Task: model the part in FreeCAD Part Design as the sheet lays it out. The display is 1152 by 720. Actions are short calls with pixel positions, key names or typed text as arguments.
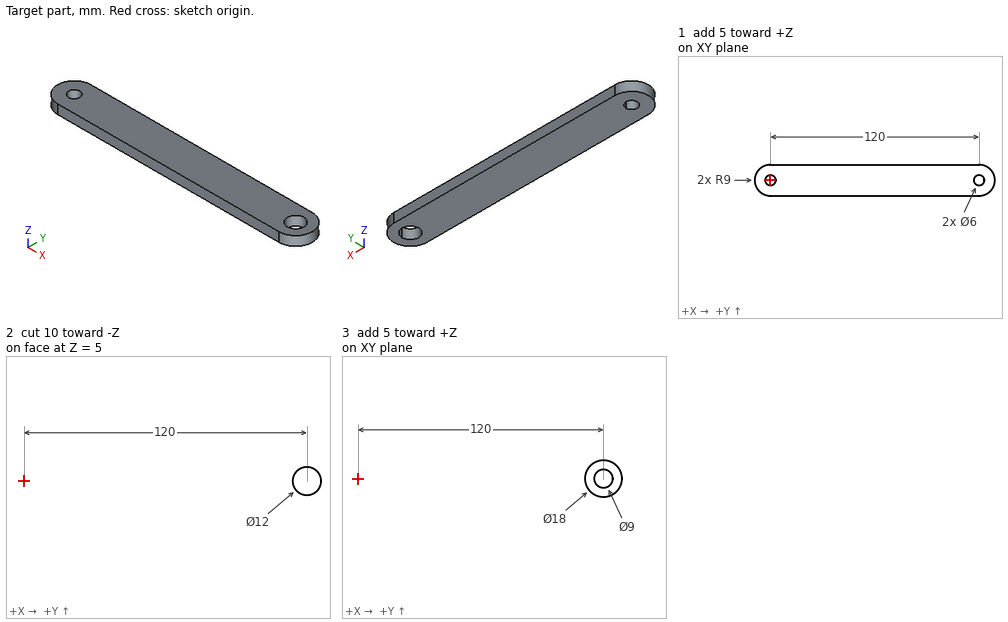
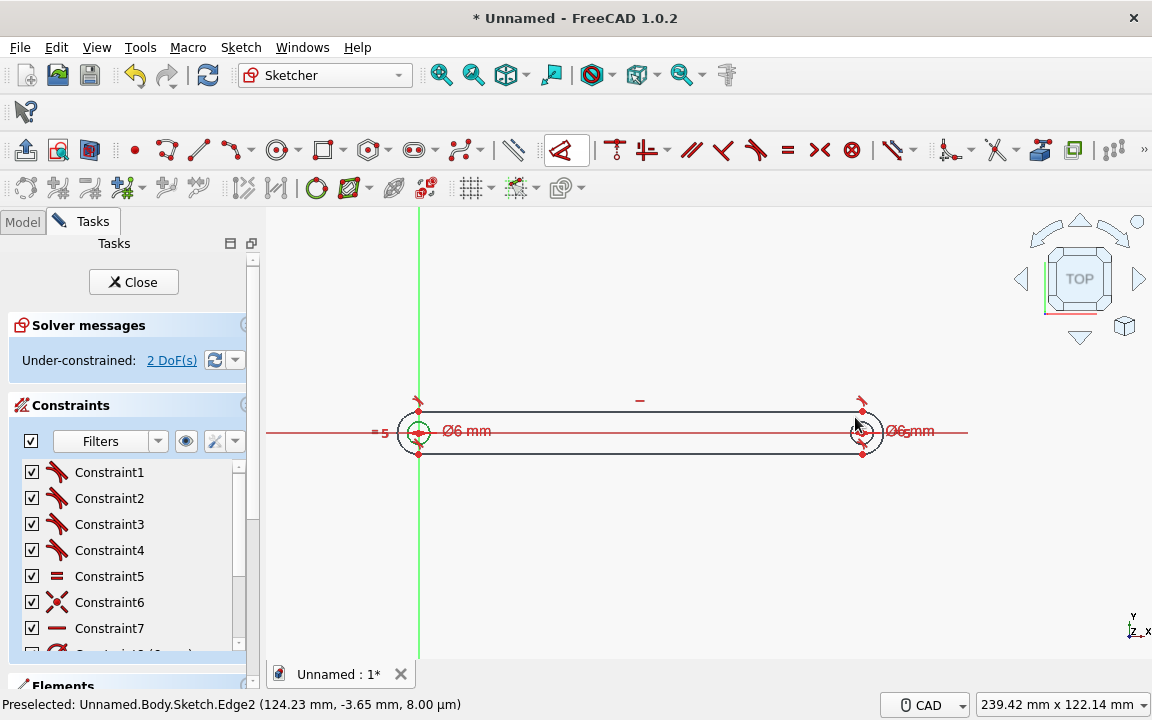
scroll(402, 421, up, 2)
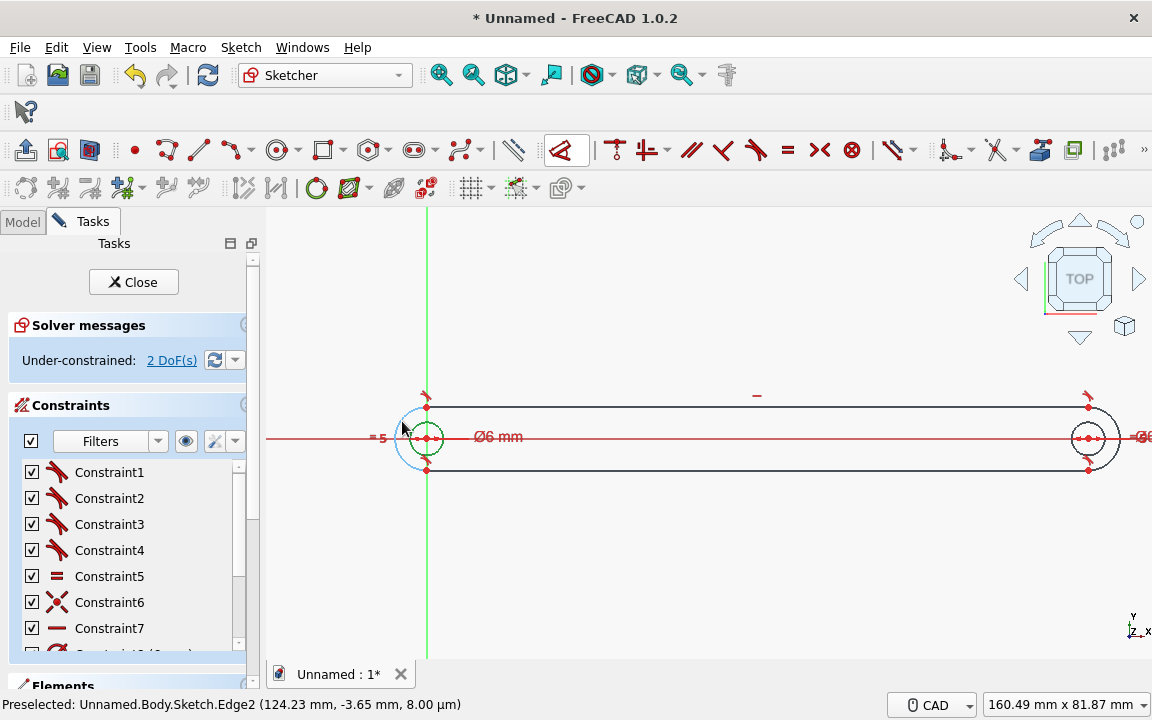
click(401, 420)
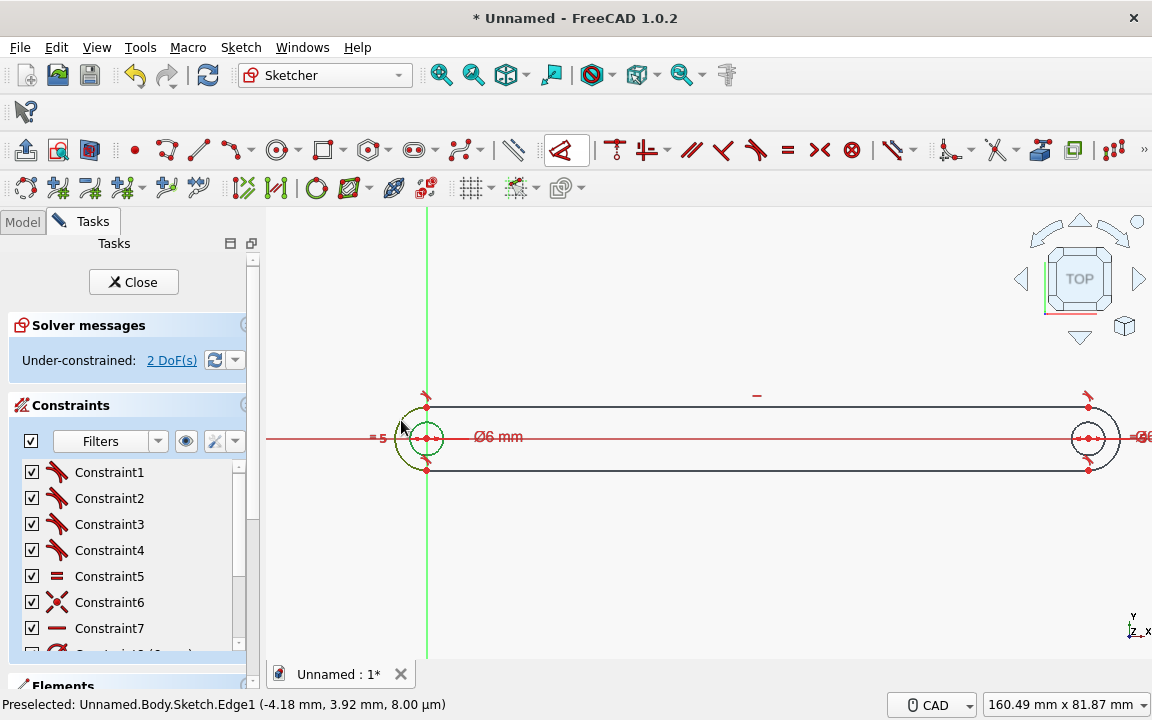
key(k)
key(r)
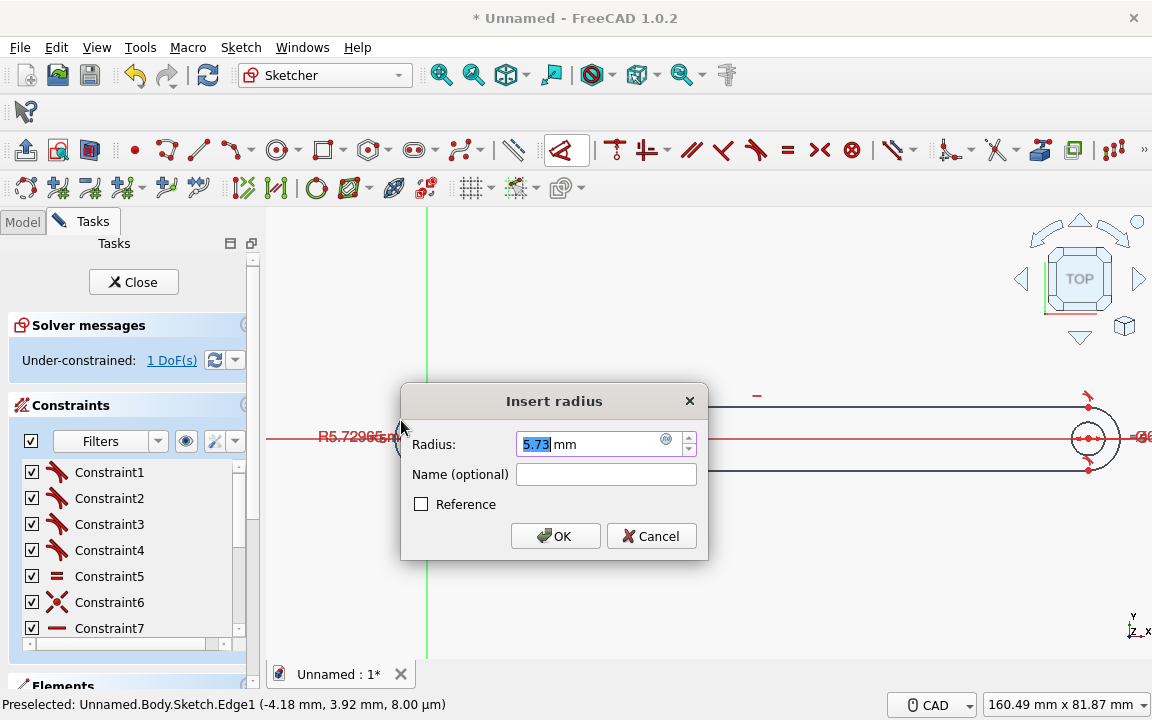
text(9)
key(Return)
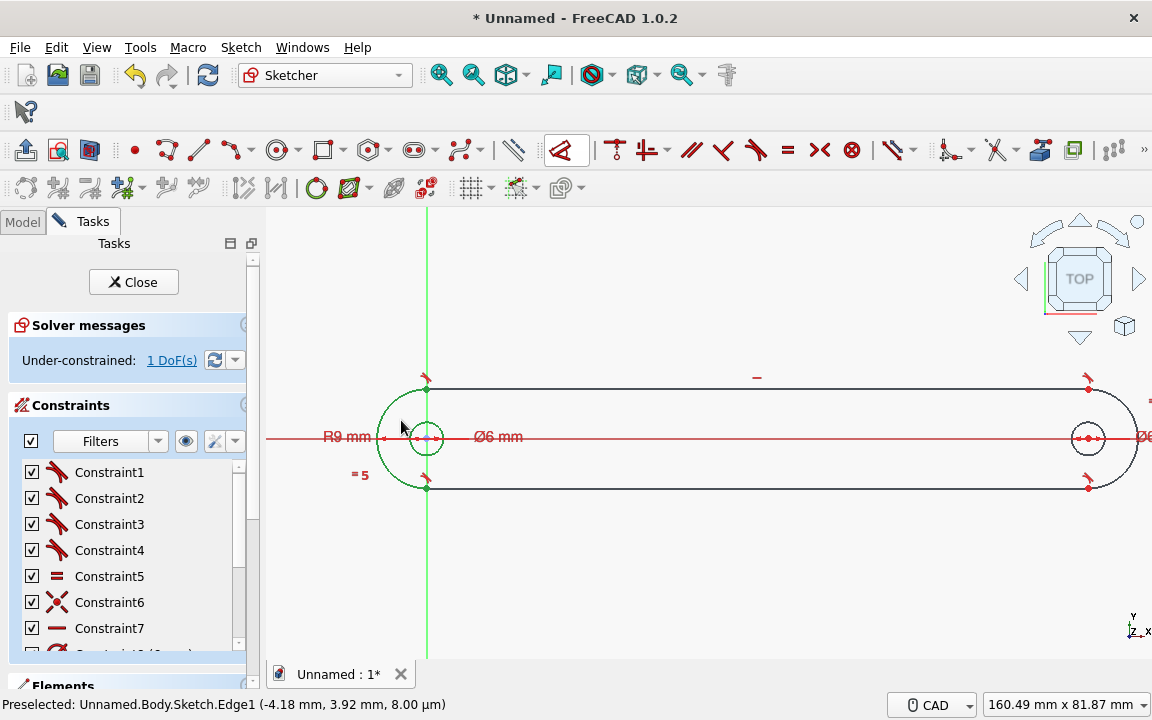
click(625, 389)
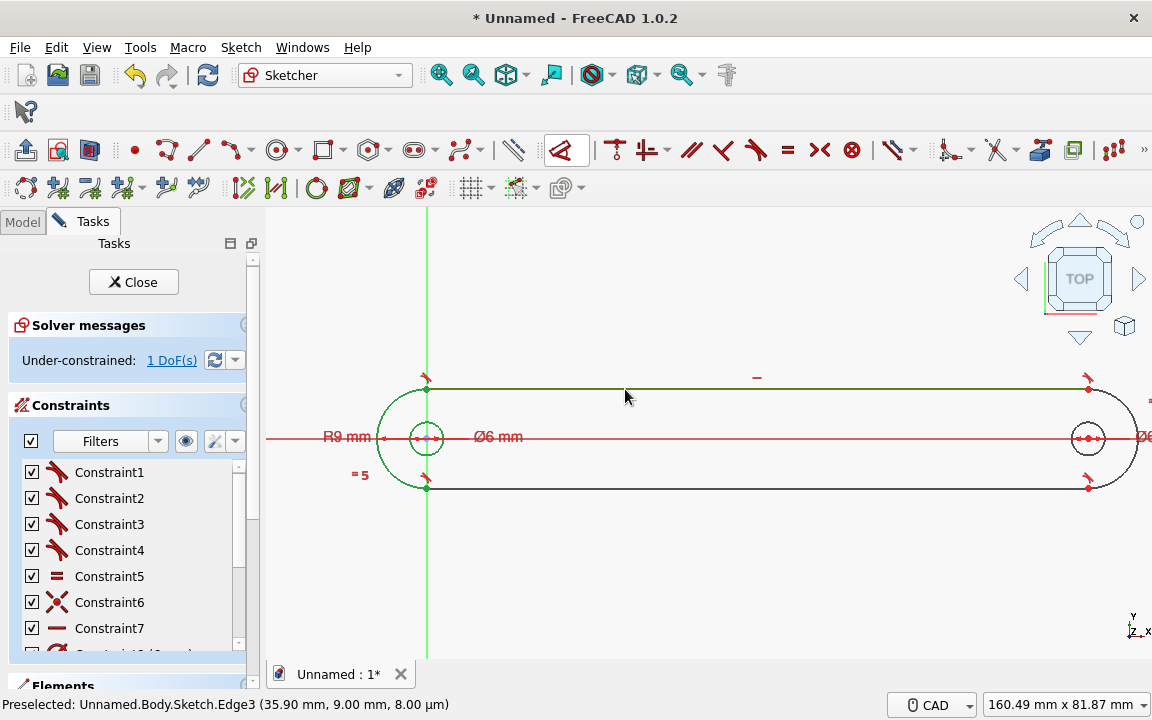
click(584, 150)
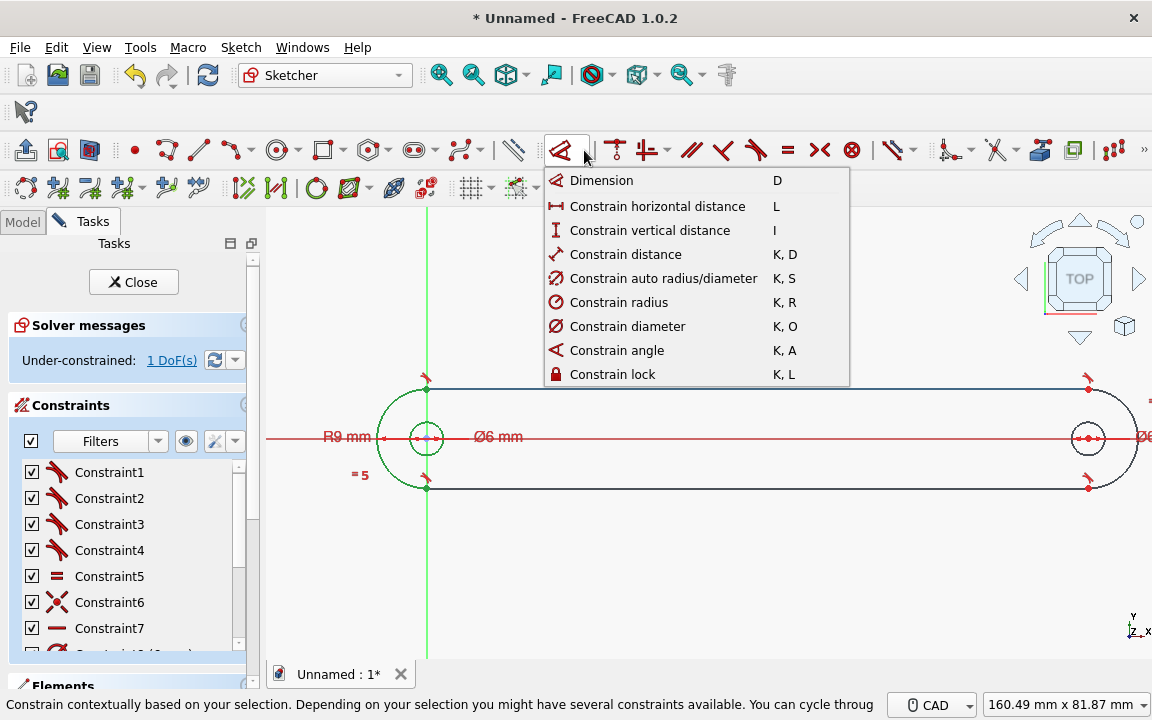
click(697, 206)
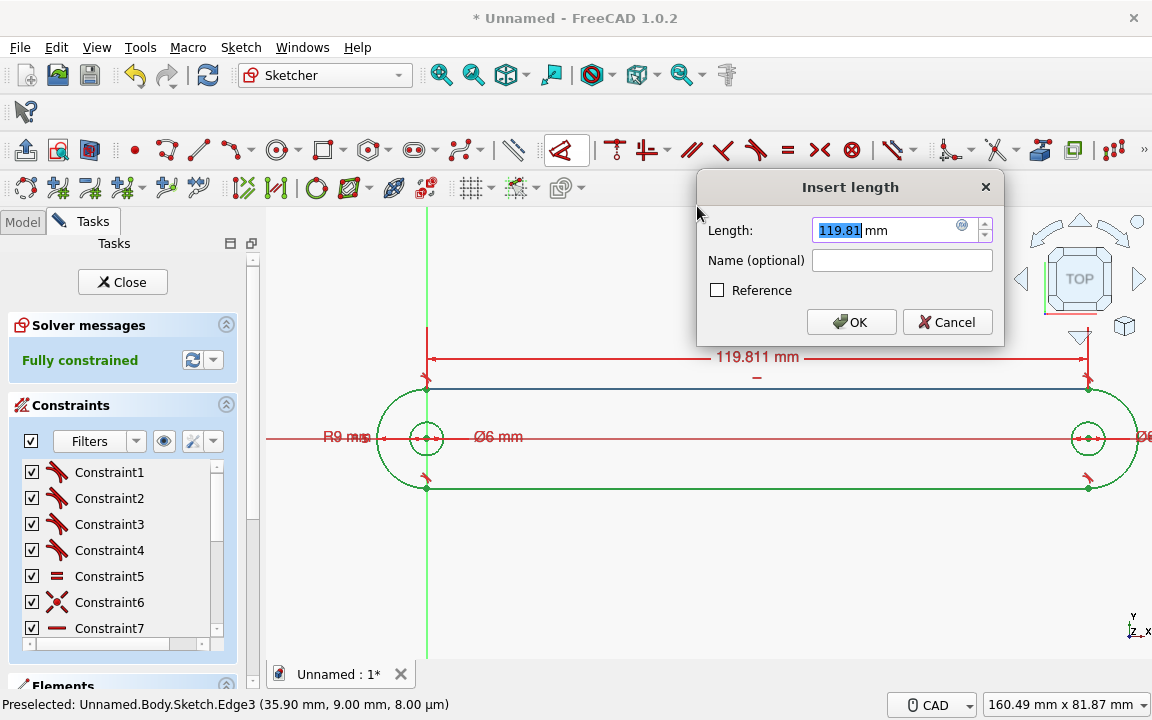
text(120)
key(Return)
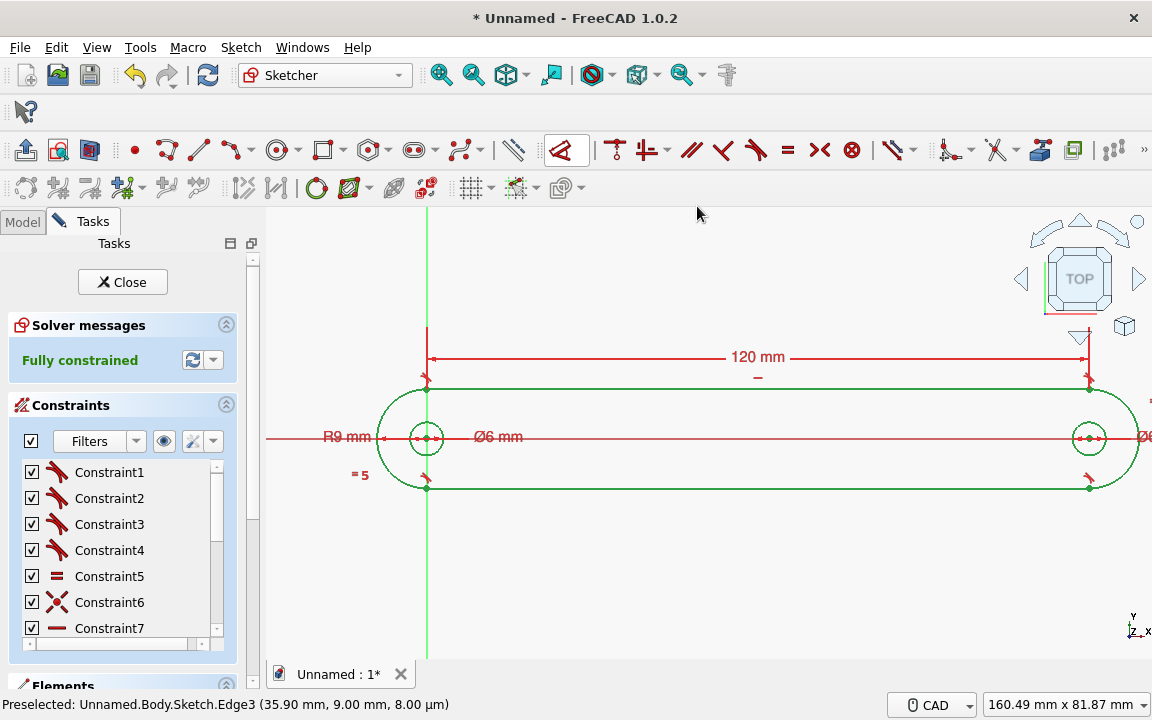
click(123, 282)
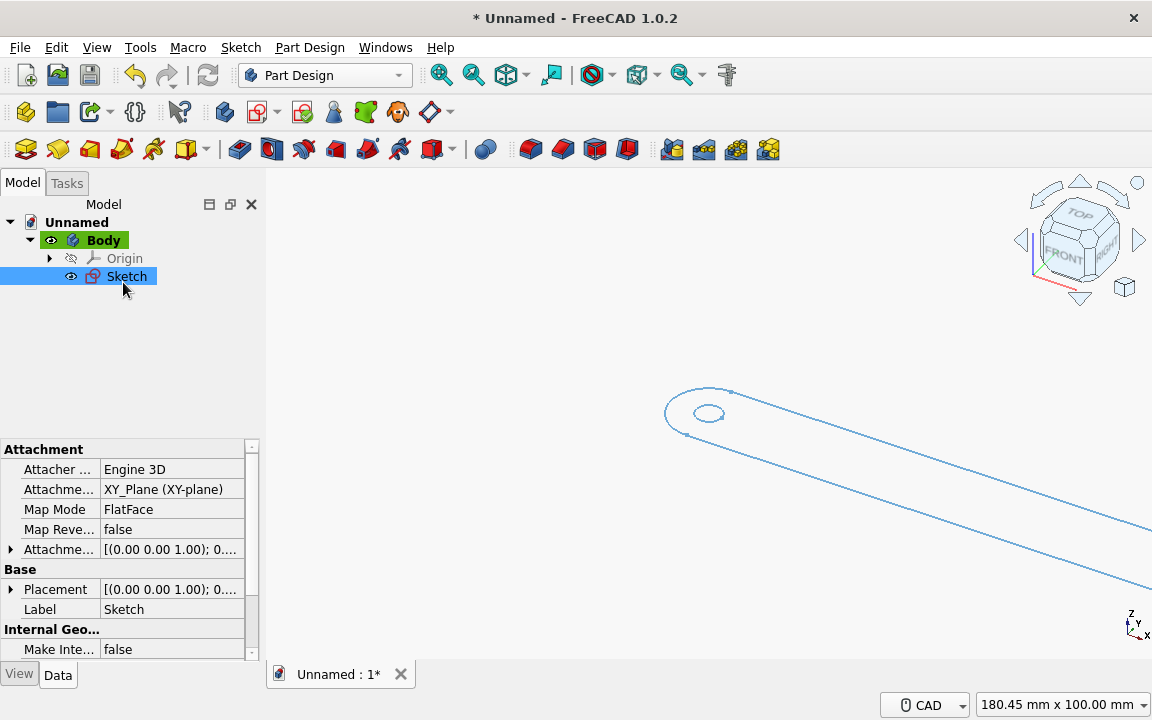
click(26, 150)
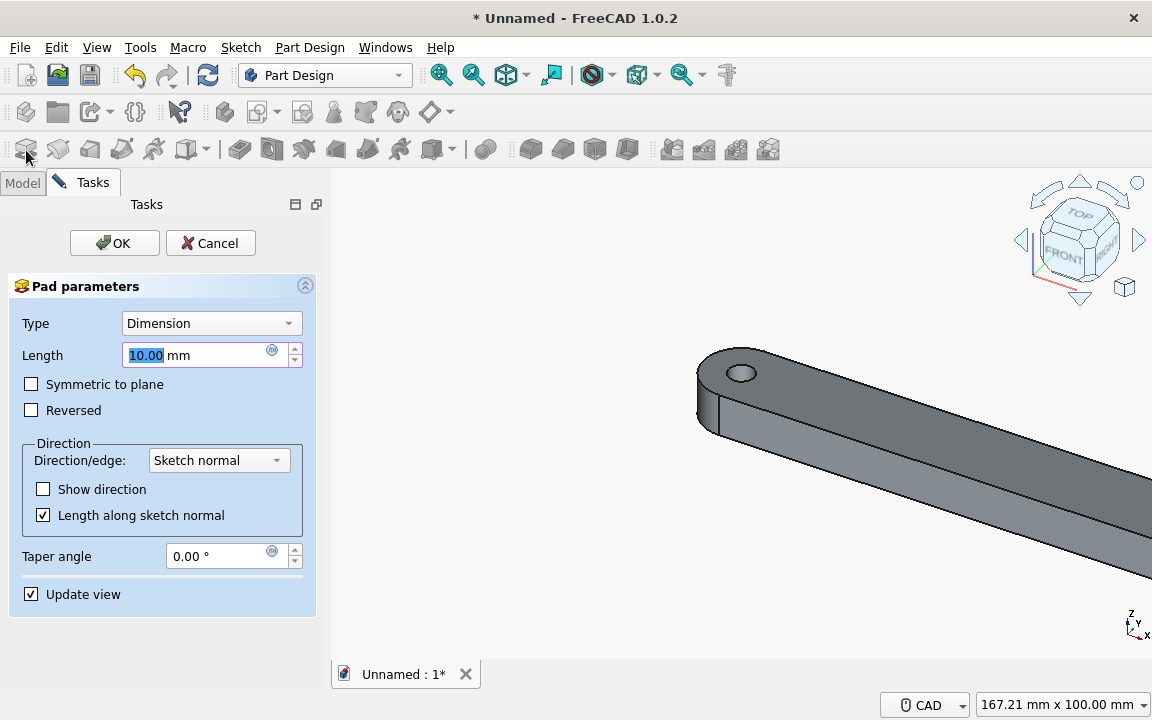
text(5)
key(Tab)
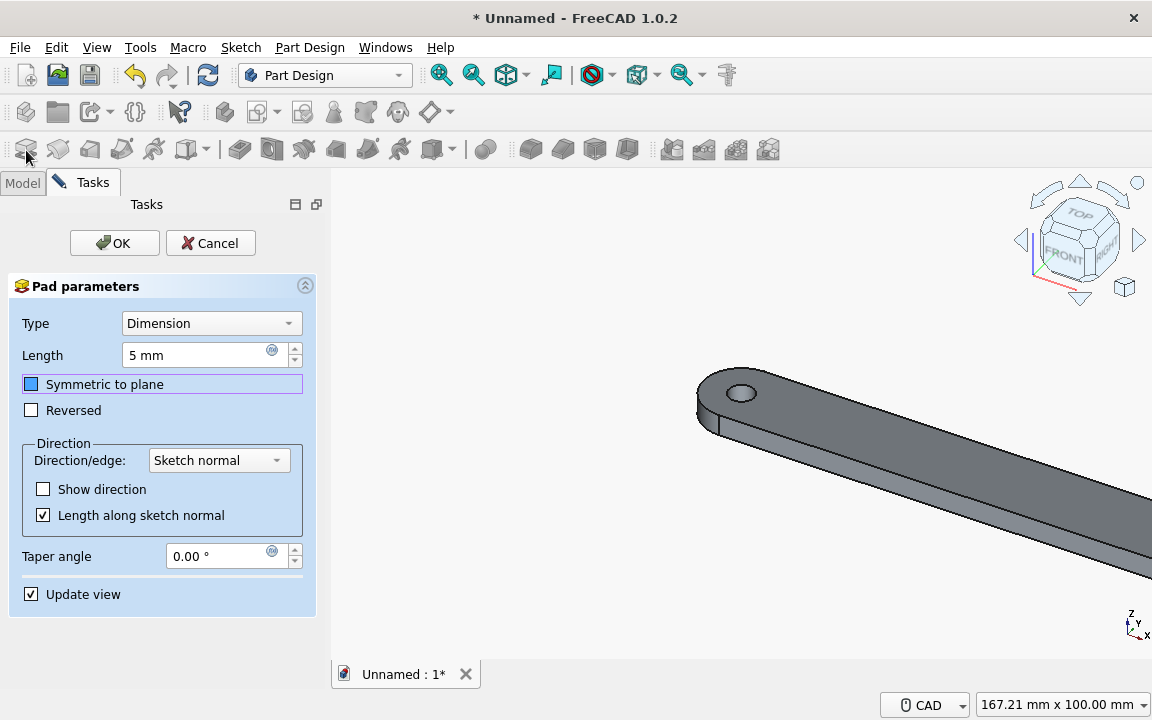
click(115, 243)